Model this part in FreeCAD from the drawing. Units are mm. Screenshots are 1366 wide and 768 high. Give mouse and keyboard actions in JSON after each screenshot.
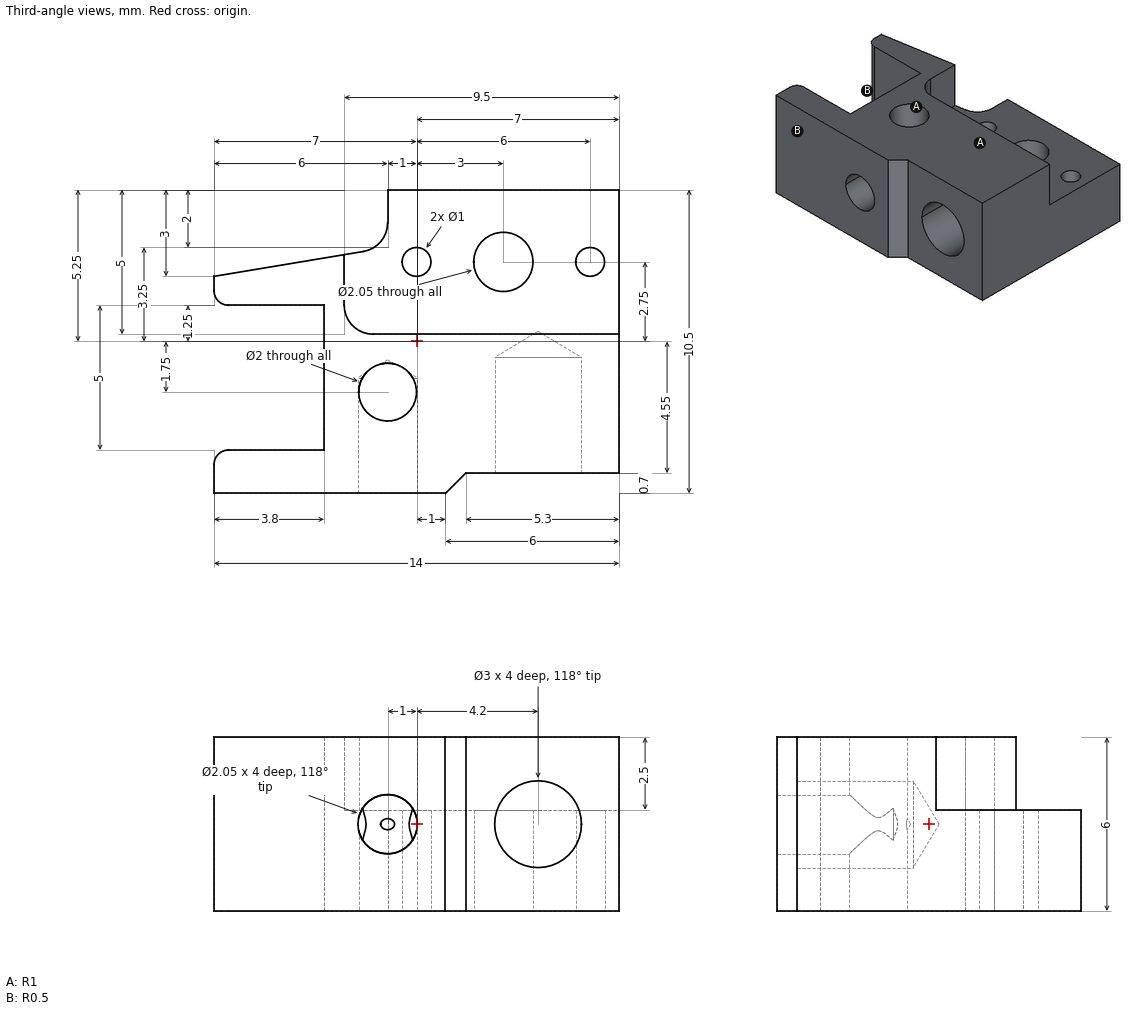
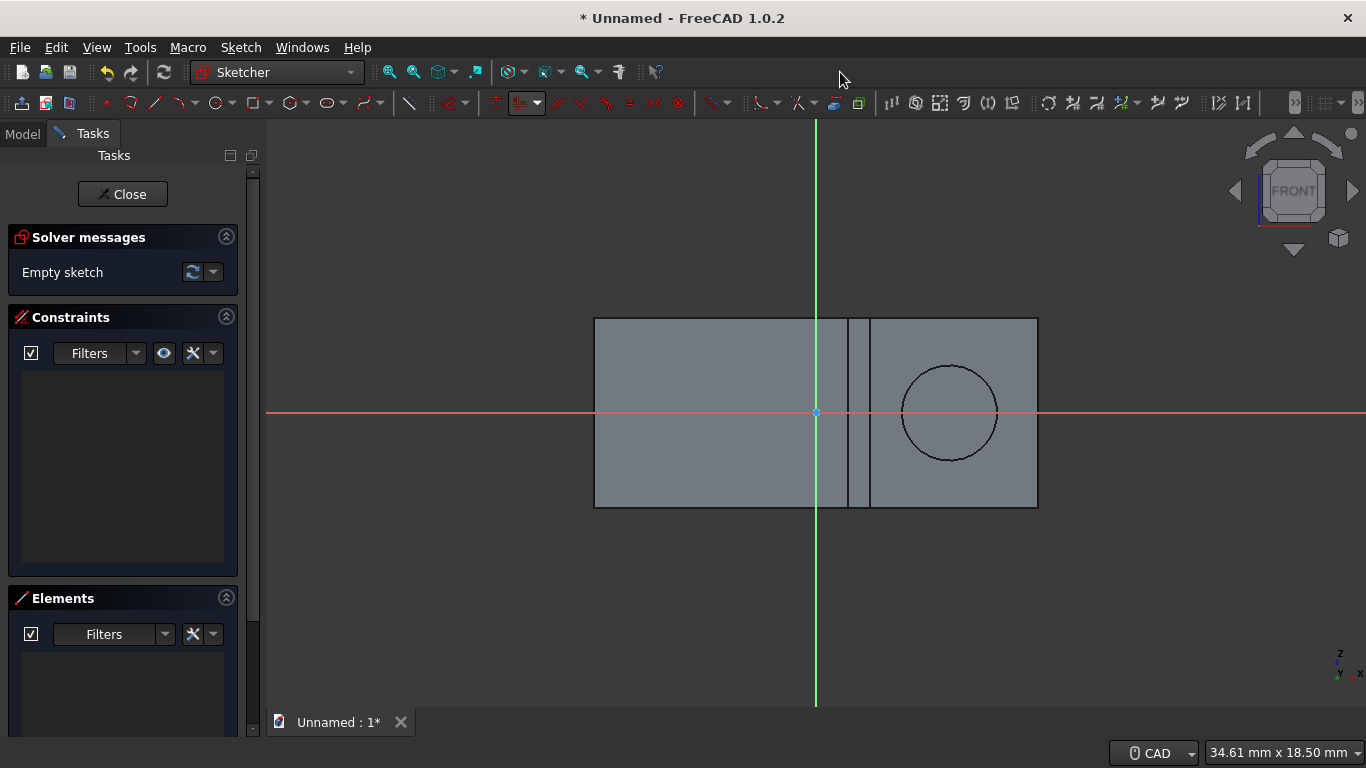
{"action": "scroll", "coordinate": [791, 413], "scroll_direction": "up", "scroll_amount": 9}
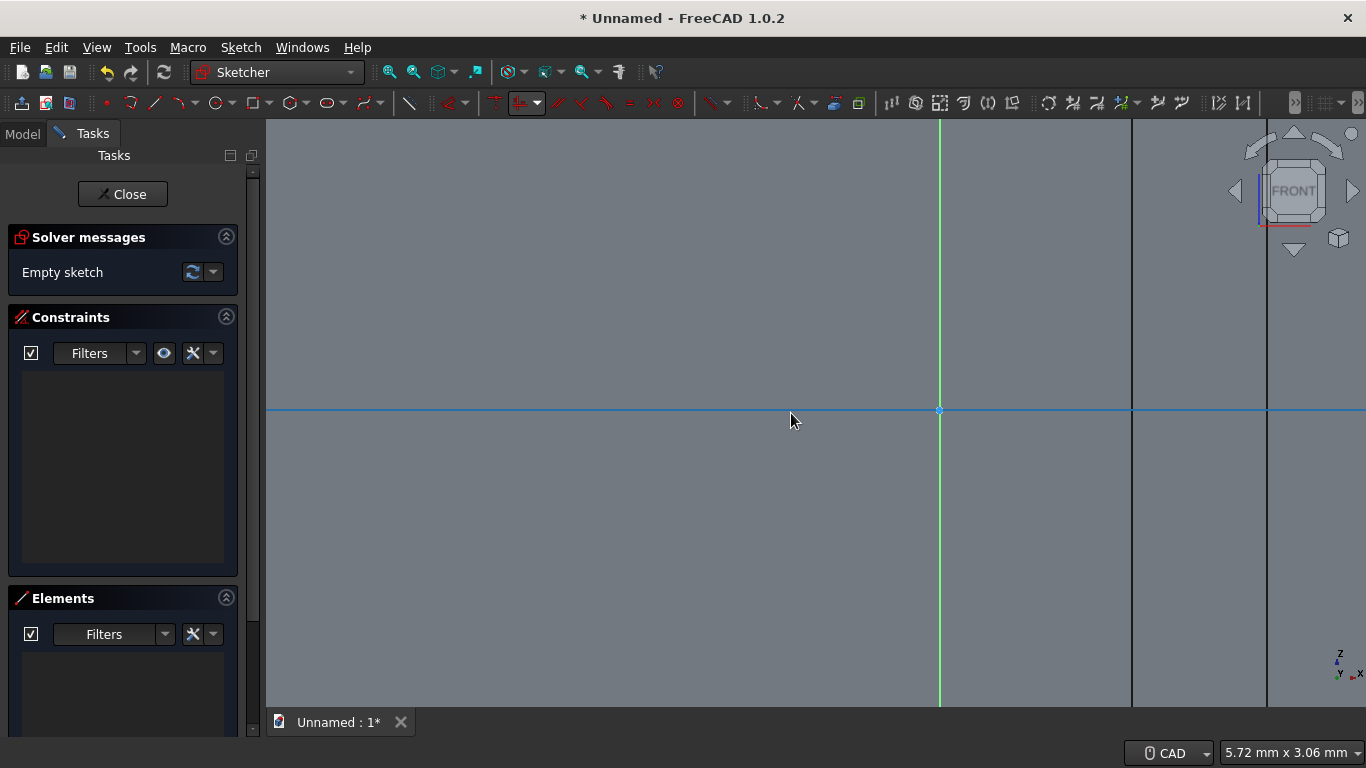
{"action": "left_click", "coordinate": [216, 104]}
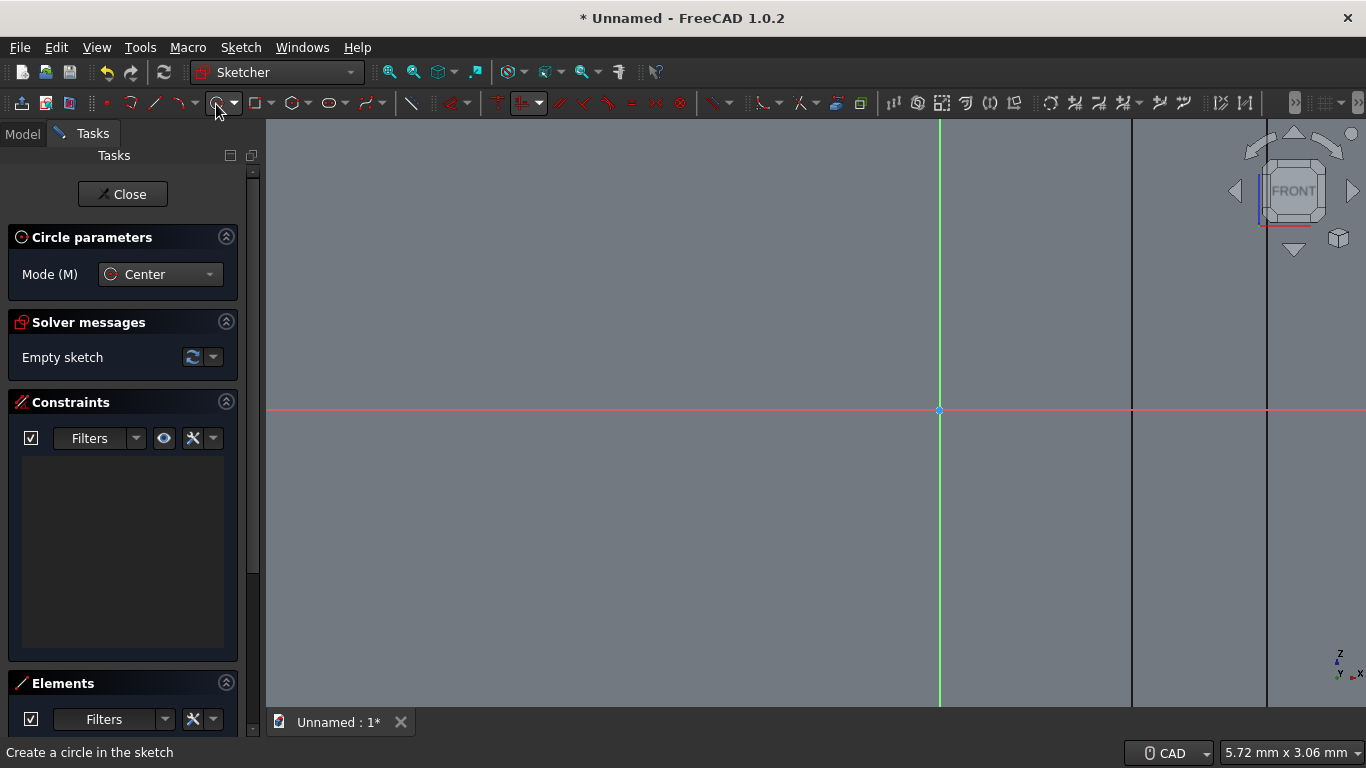
{"action": "left_click", "coordinate": [748, 410]}
{"action": "left_click", "coordinate": [887, 271]}
{"action": "key", "text": "Escape"}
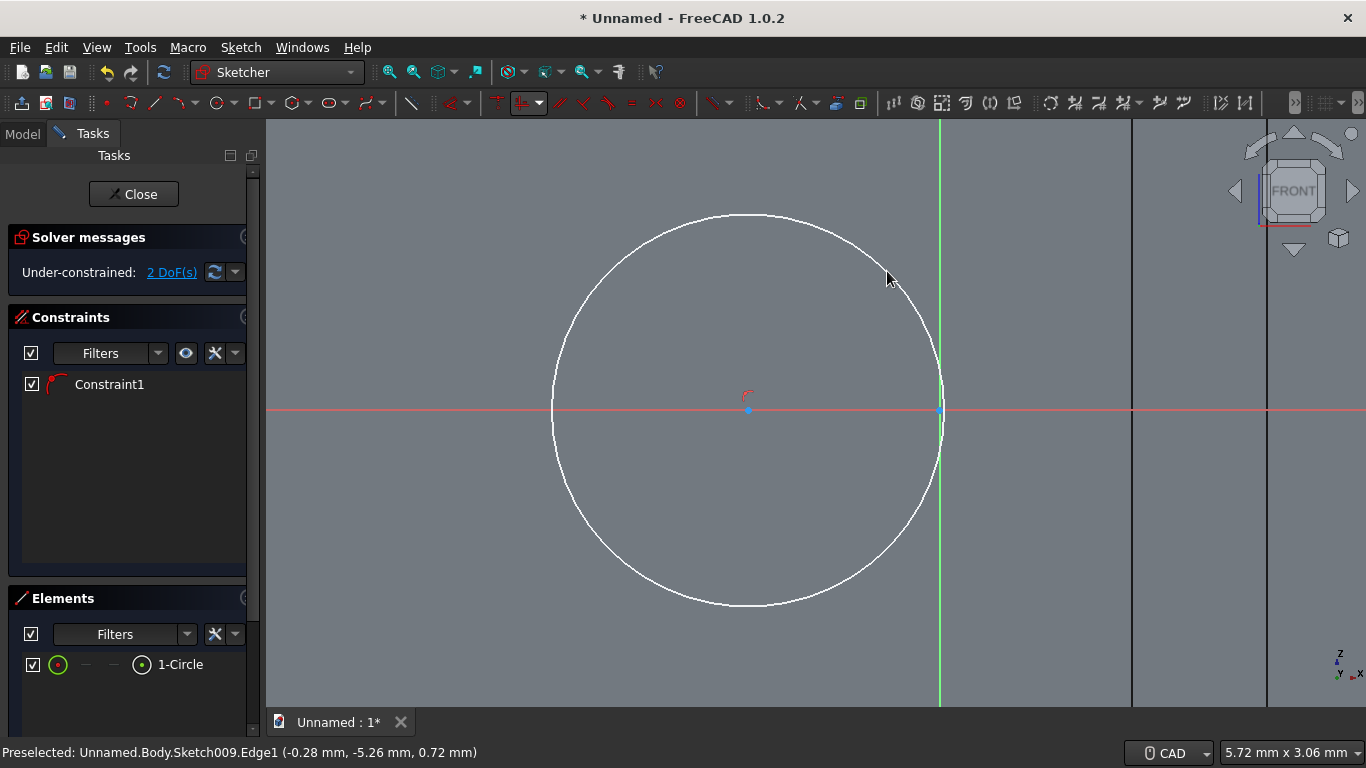
{"action": "left_click", "coordinate": [450, 104]}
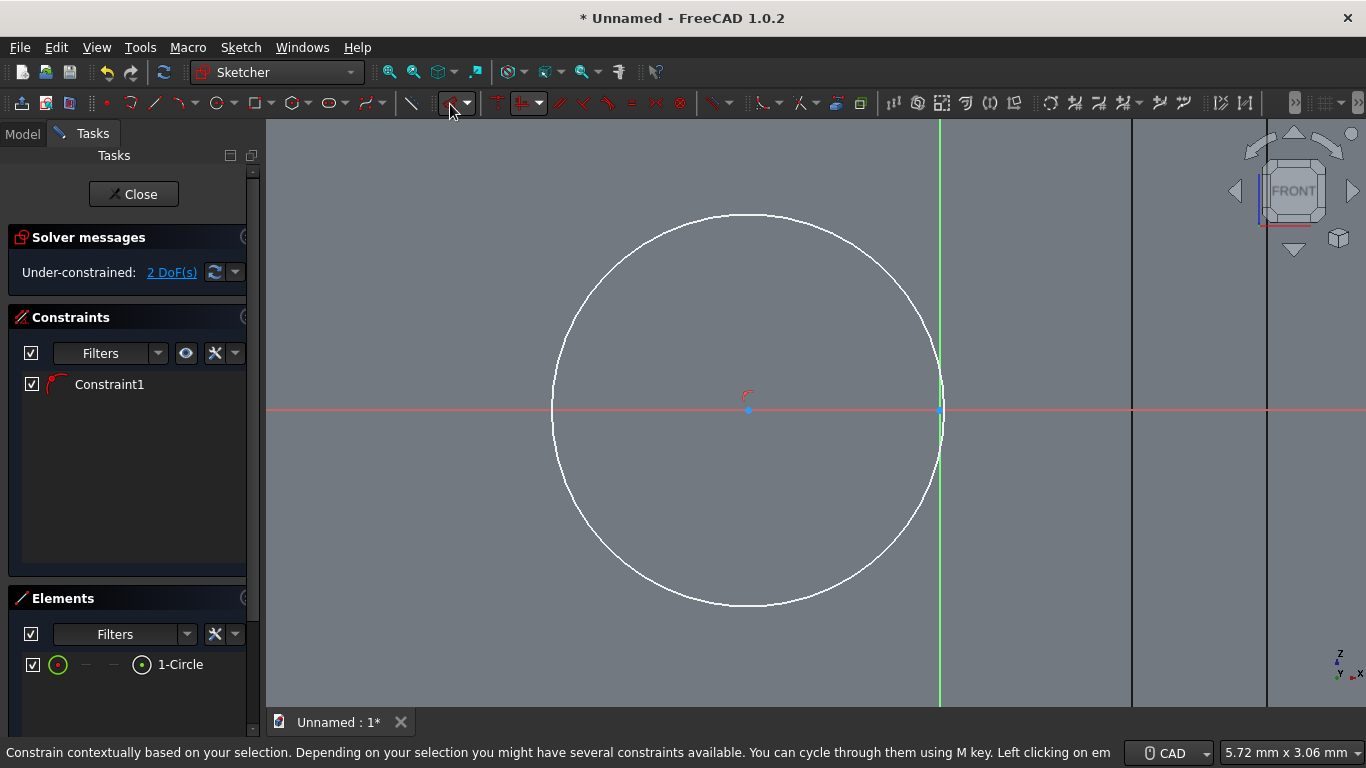
{"action": "left_click", "coordinate": [886, 271]}
{"action": "left_click", "coordinate": [909, 248]}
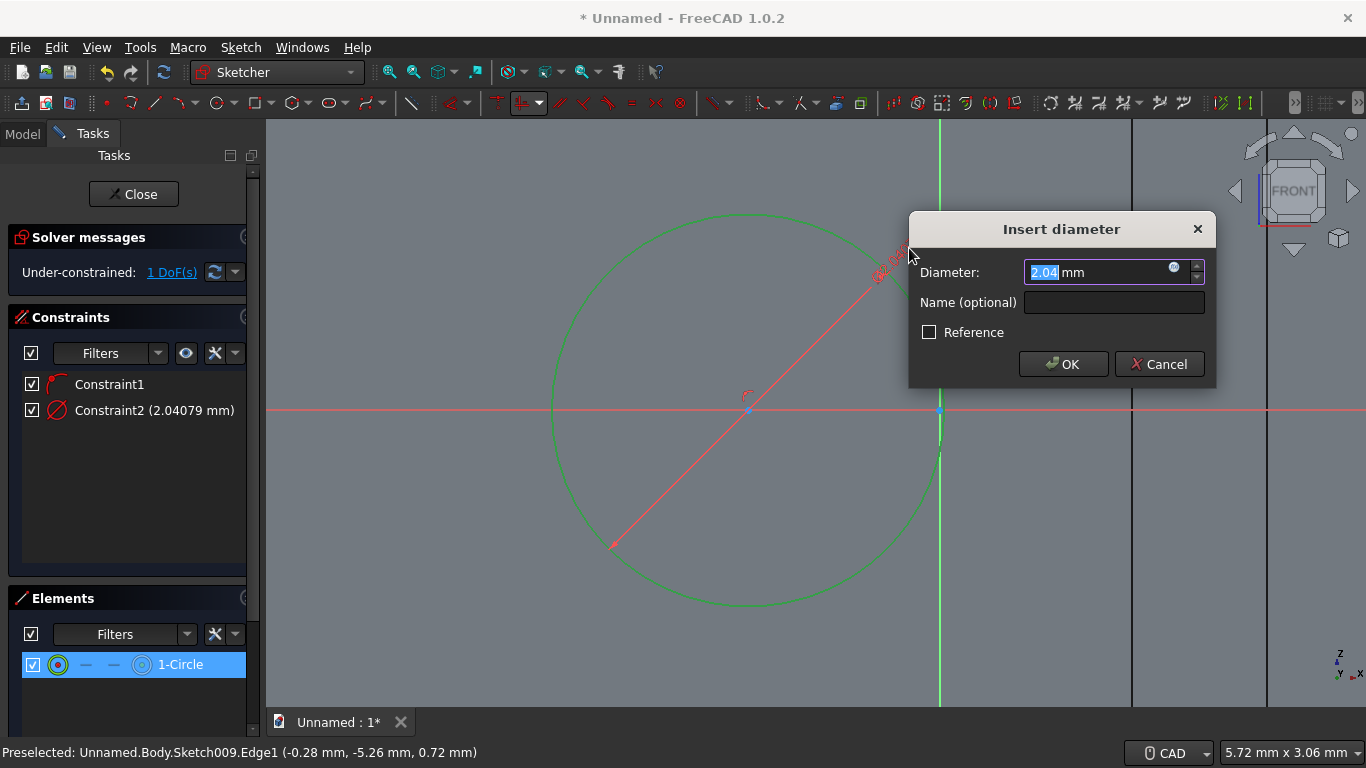
{"action": "type", "text": "2.05"}
{"action": "key", "text": "Return"}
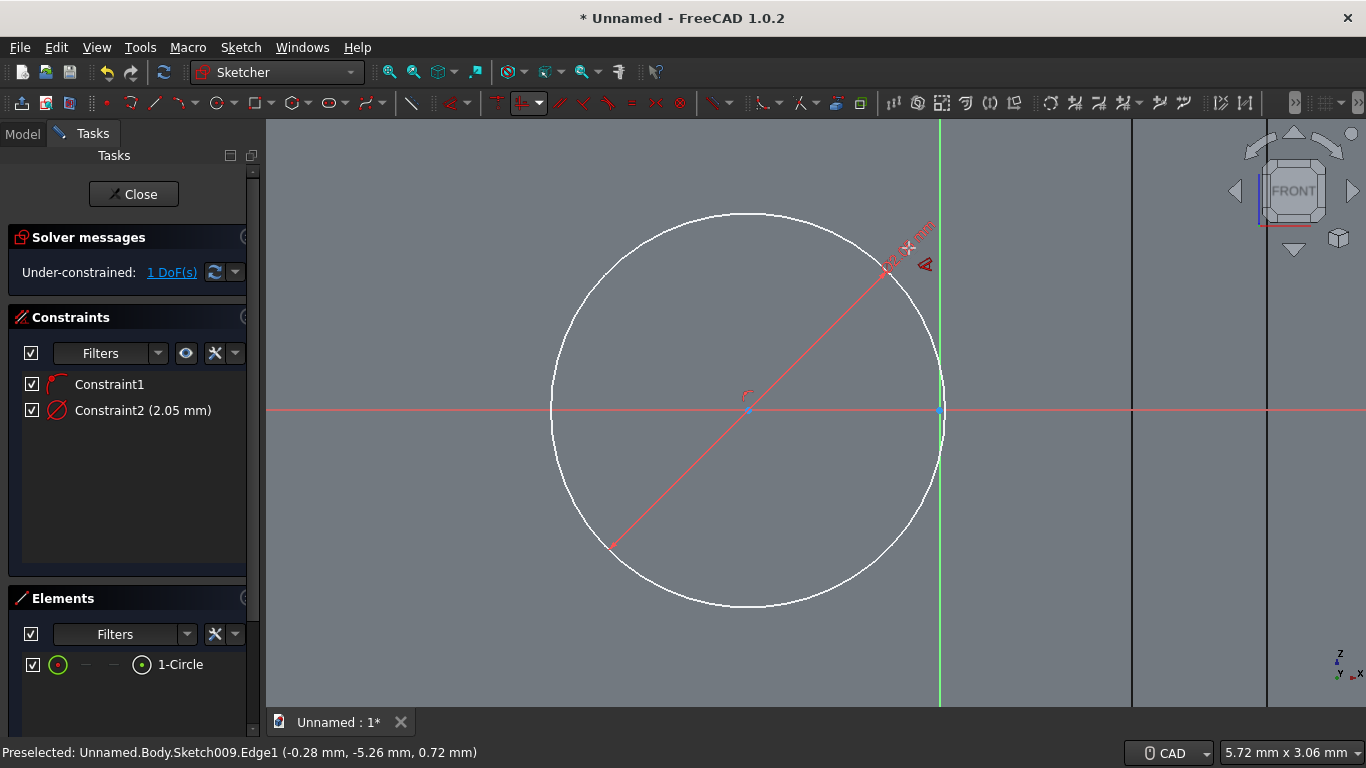
{"action": "left_click", "coordinate": [748, 410]}
{"action": "left_click", "coordinate": [844, 444]}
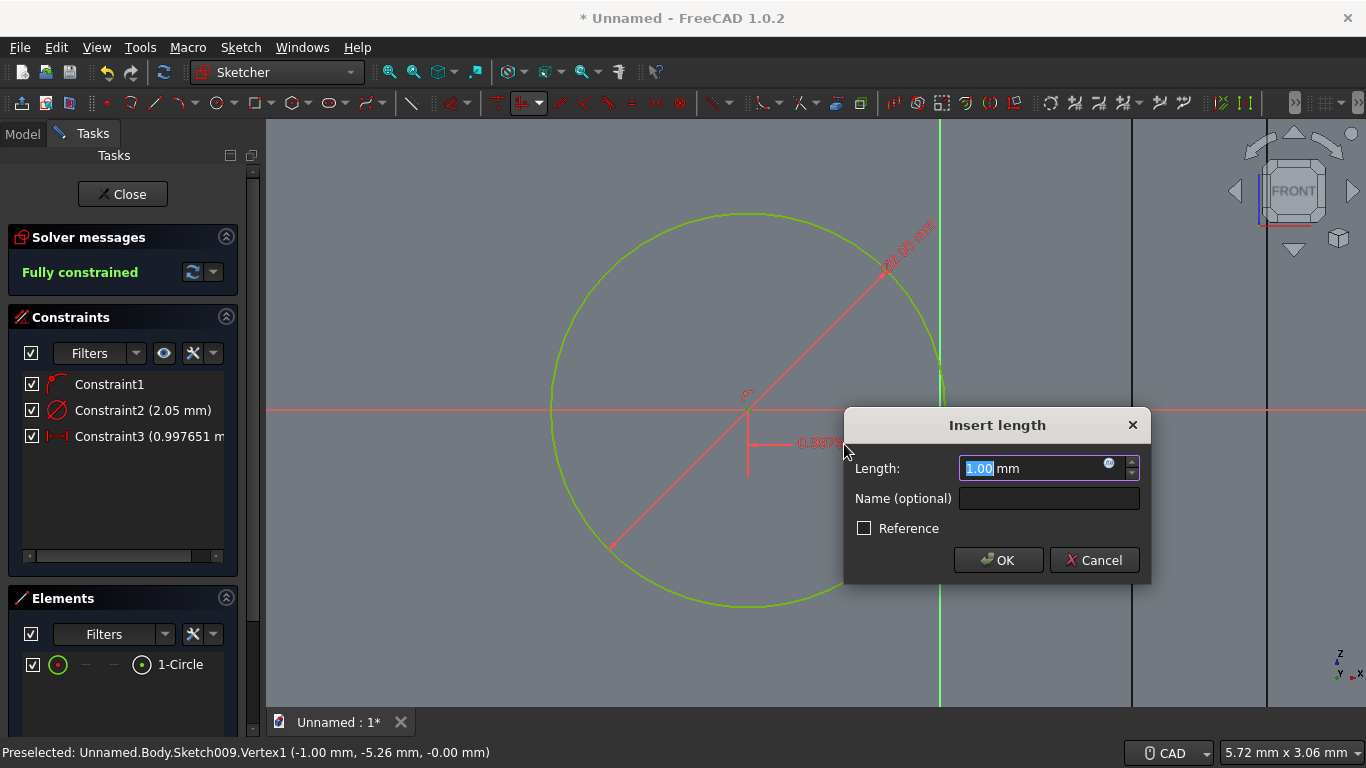
{"action": "type", "text": "1"}
{"action": "key", "text": "Return"}
{"action": "key", "text": "Escape"}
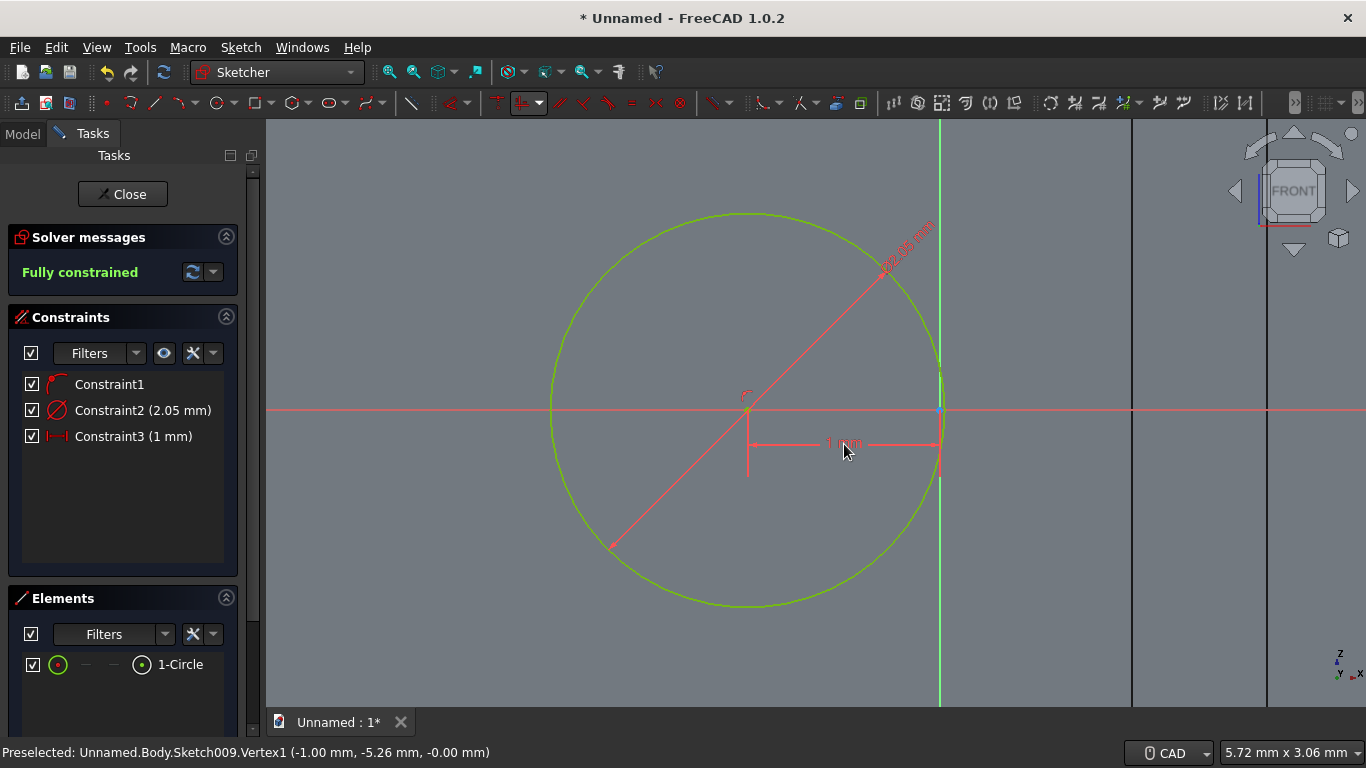
{"action": "left_click", "coordinate": [123, 194]}